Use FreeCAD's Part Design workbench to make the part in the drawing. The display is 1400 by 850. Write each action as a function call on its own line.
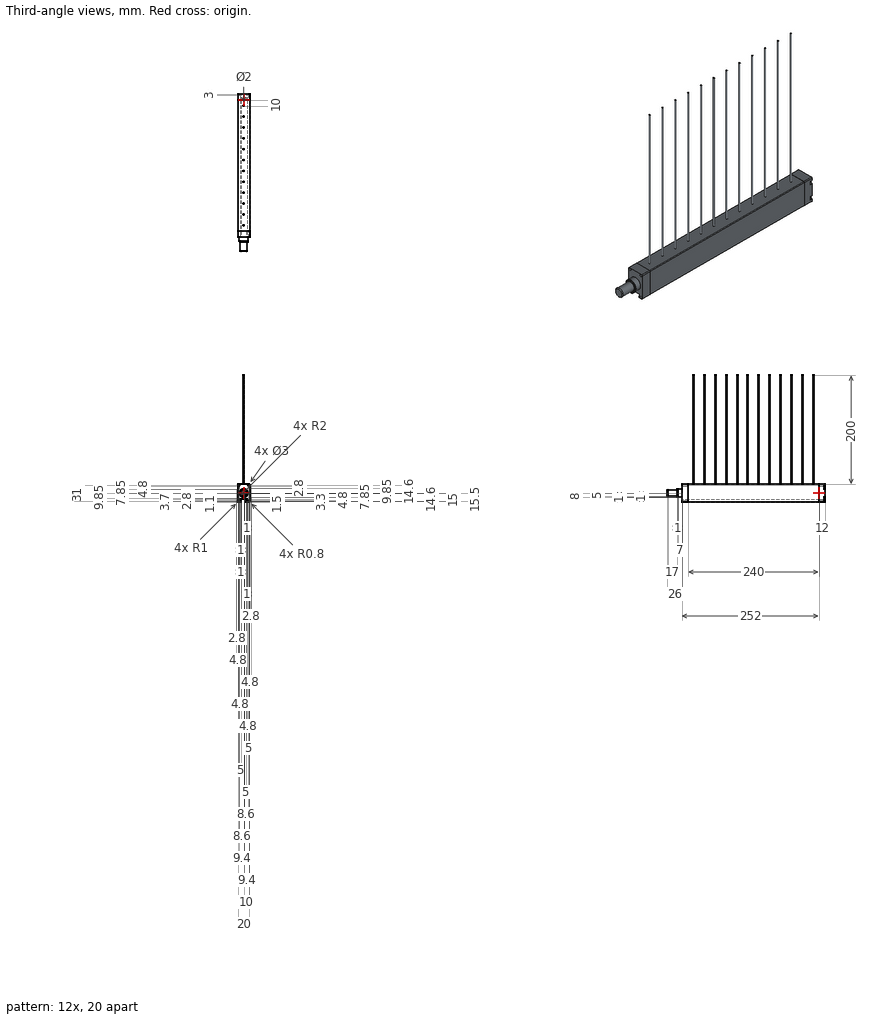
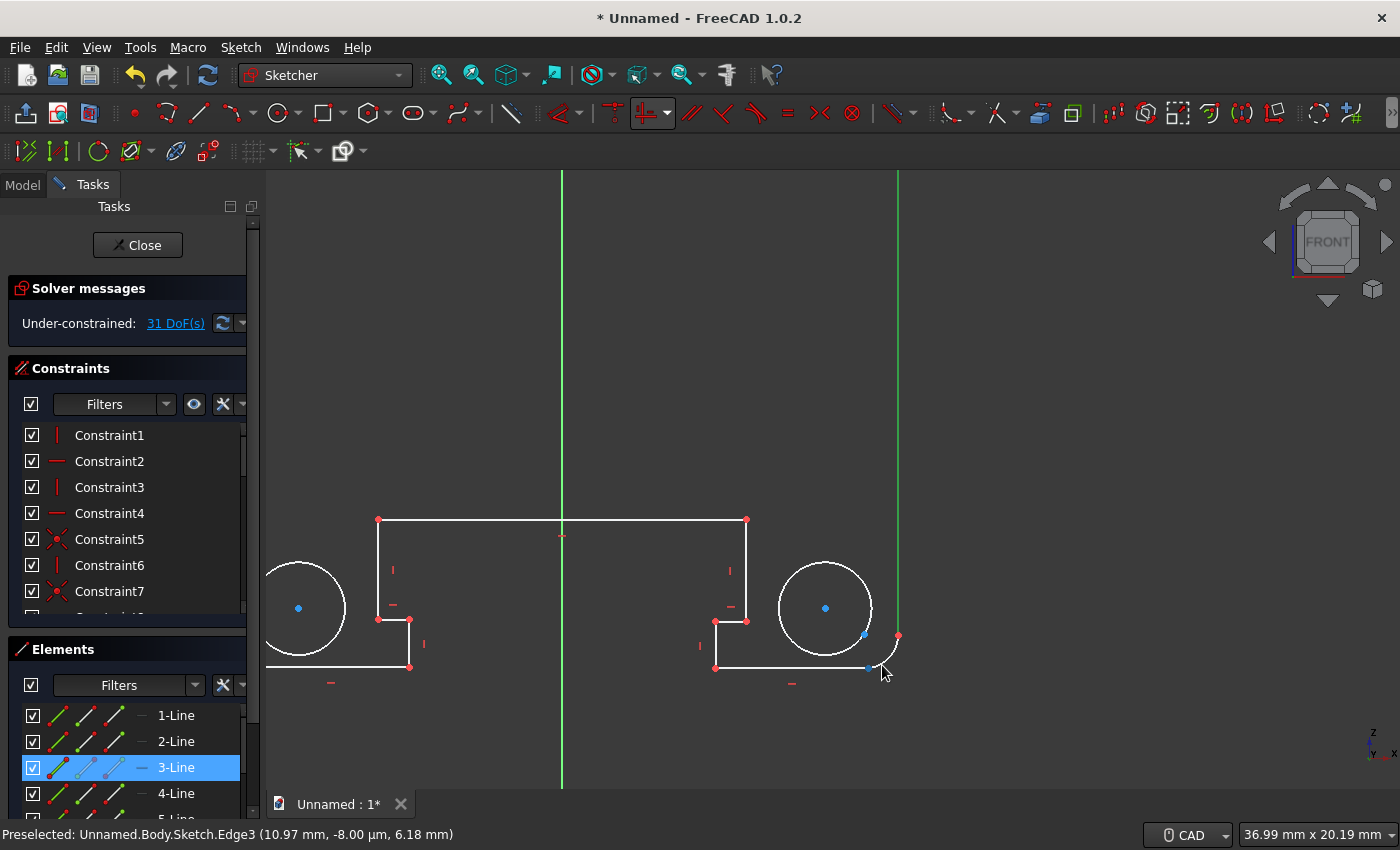
click(882, 664)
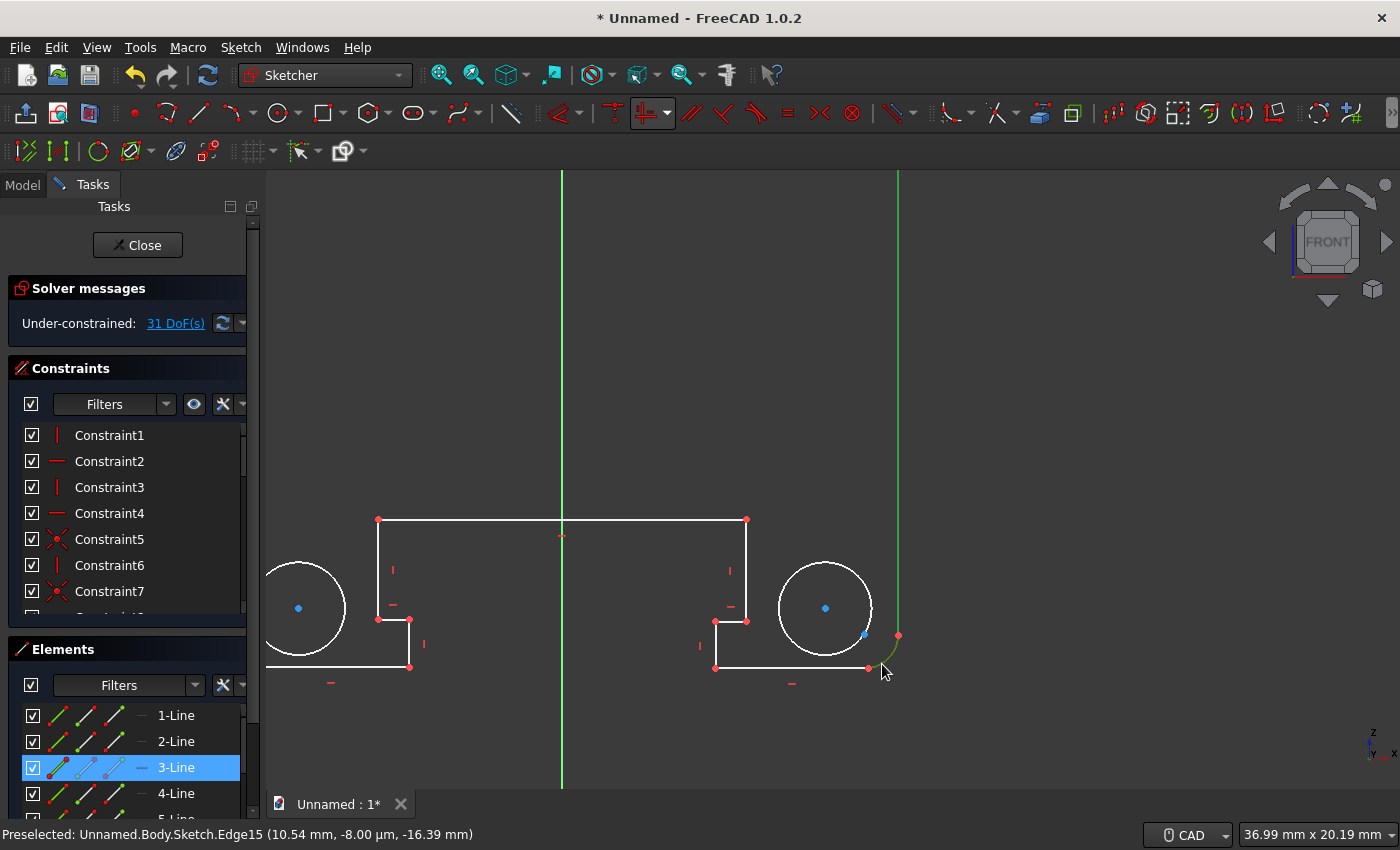
click(756, 114)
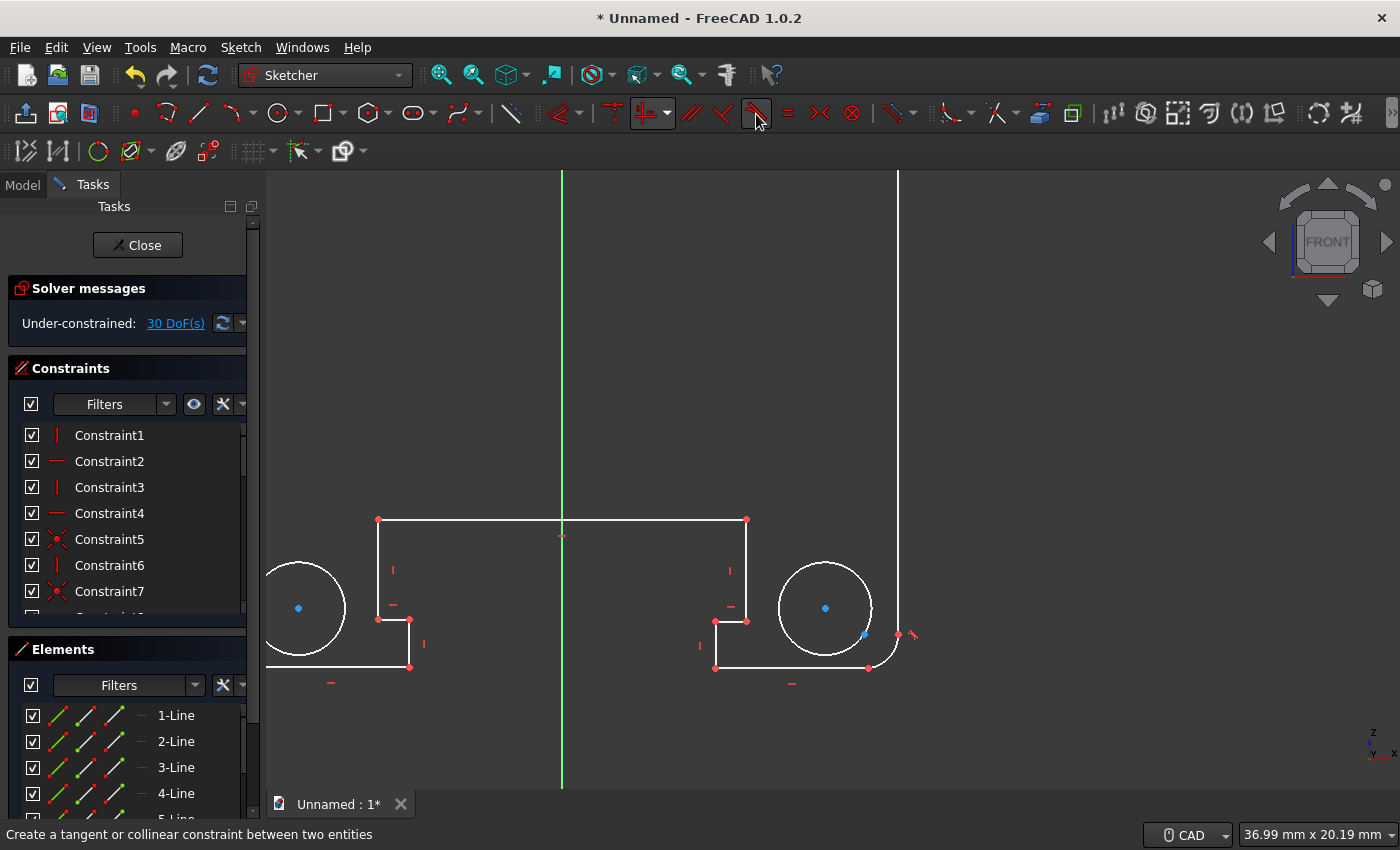
click(823, 668)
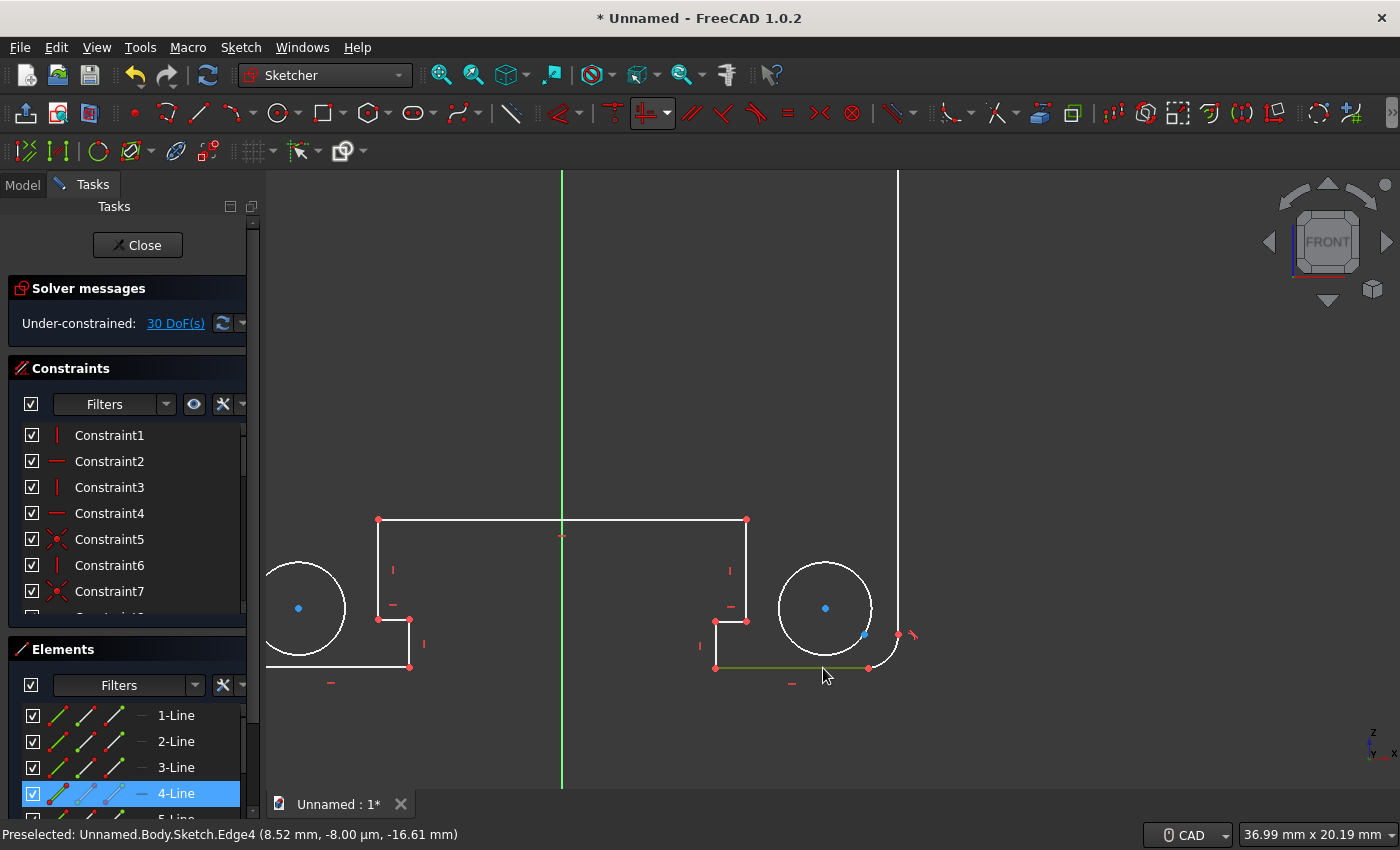
click(882, 663)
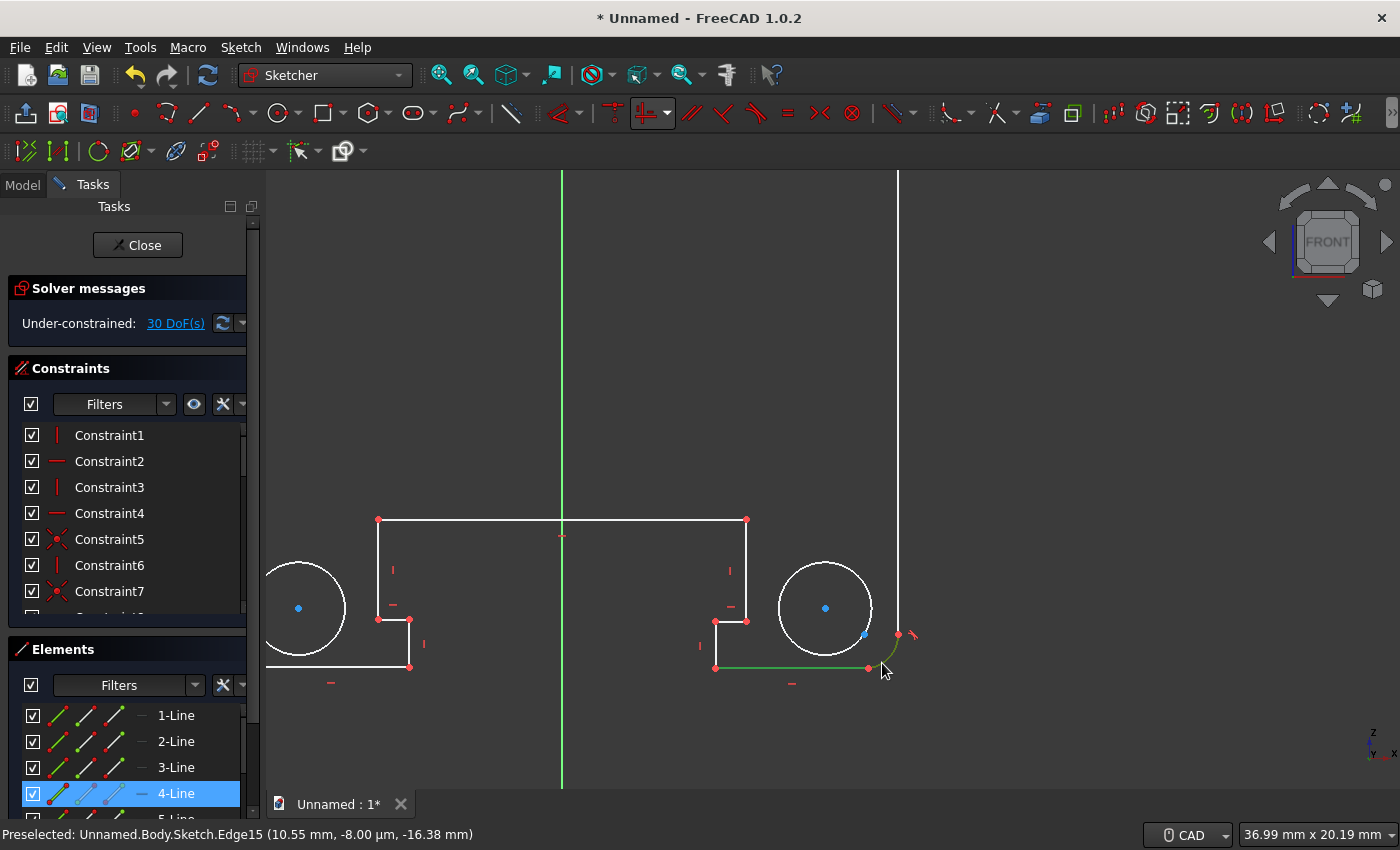
click(756, 114)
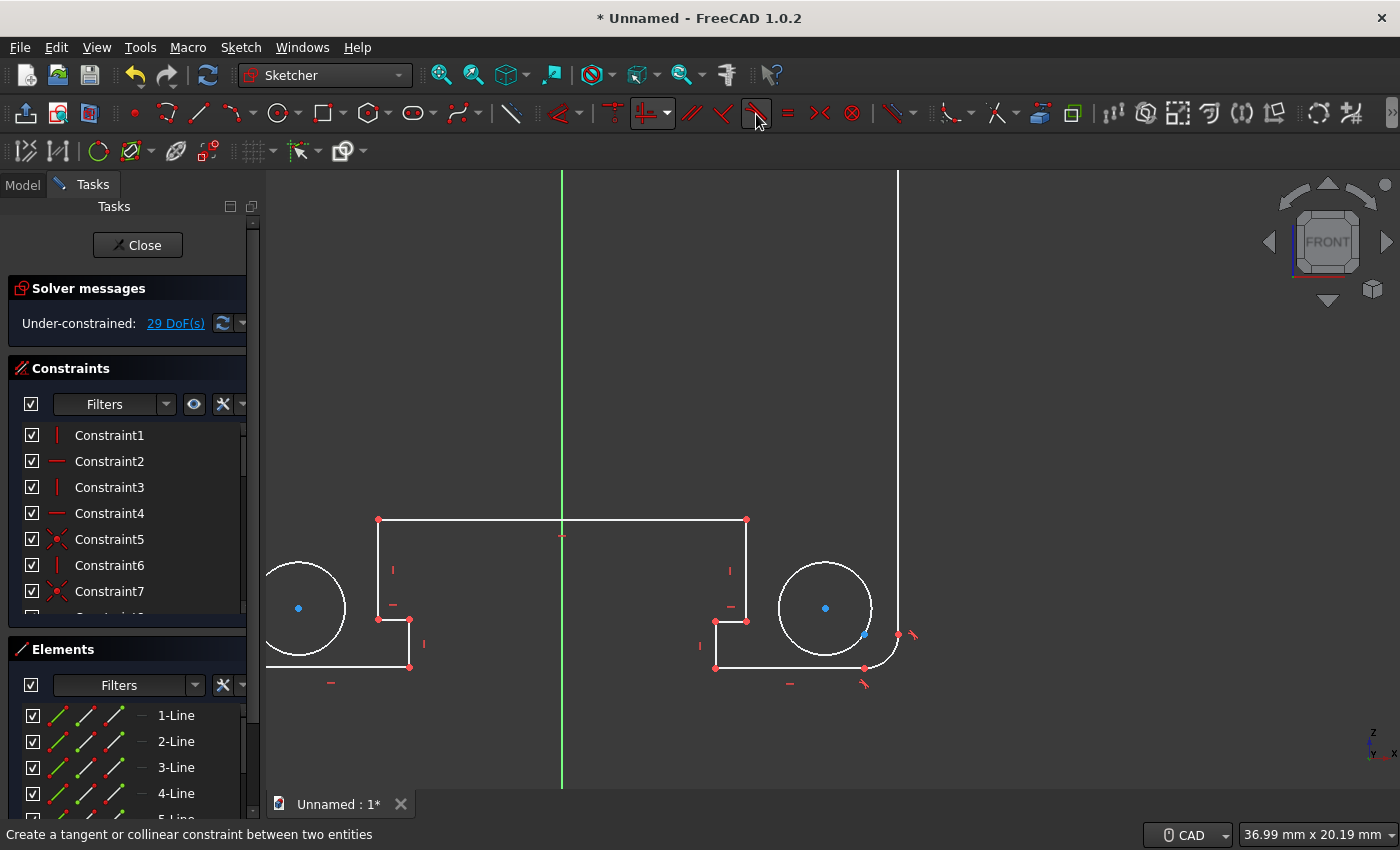
click(363, 667)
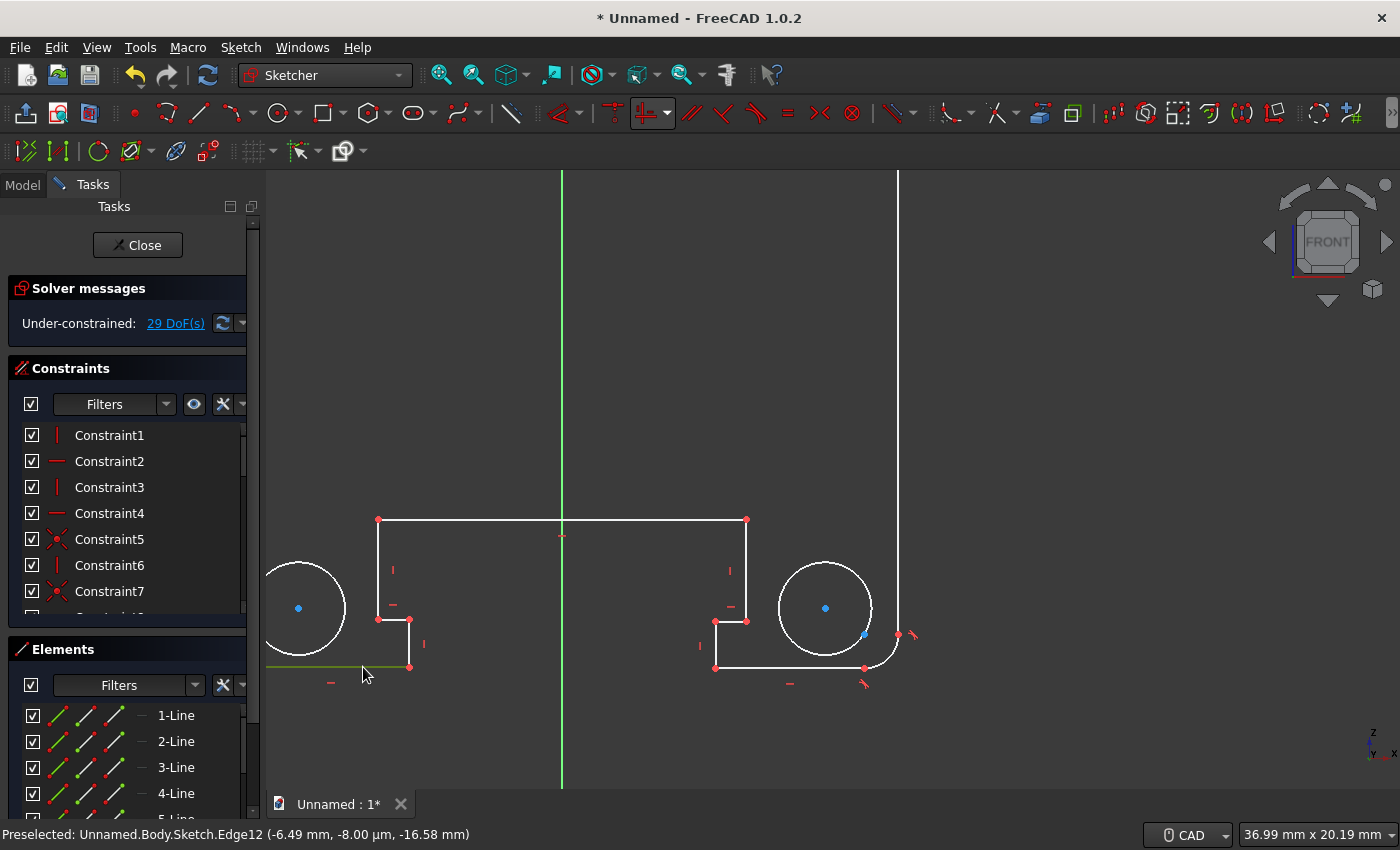
scroll(882, 666, down, 5)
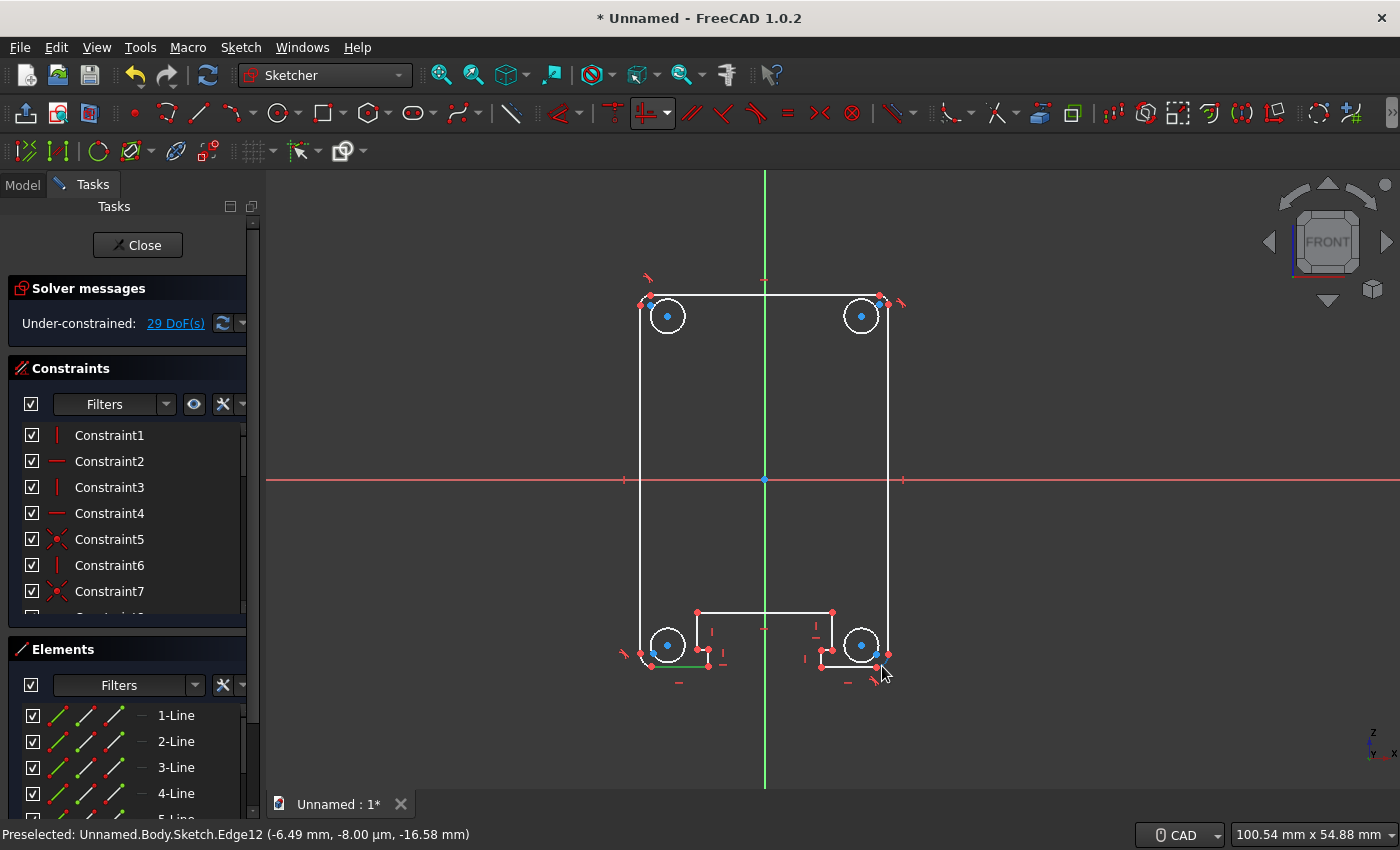
scroll(641, 659, up, 5)